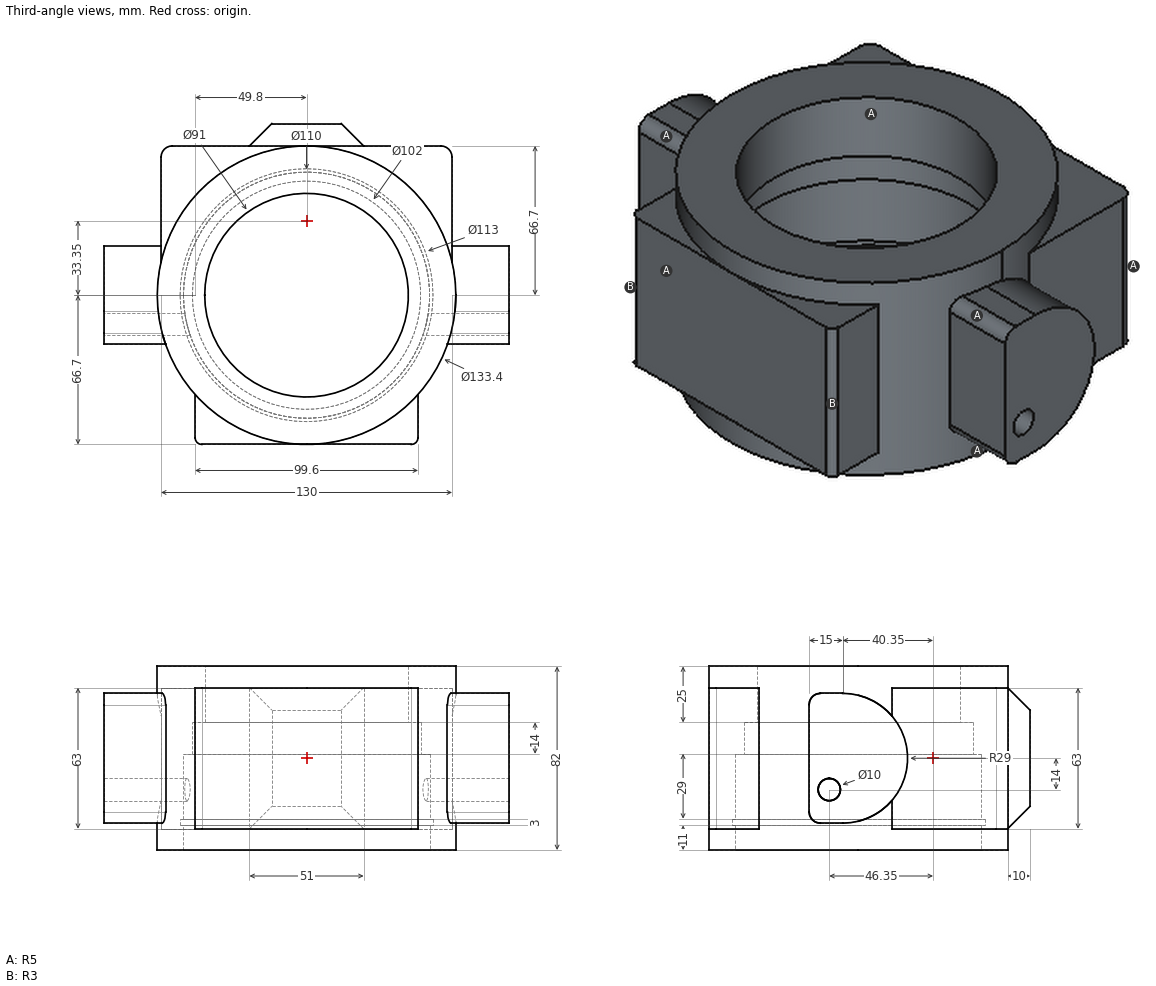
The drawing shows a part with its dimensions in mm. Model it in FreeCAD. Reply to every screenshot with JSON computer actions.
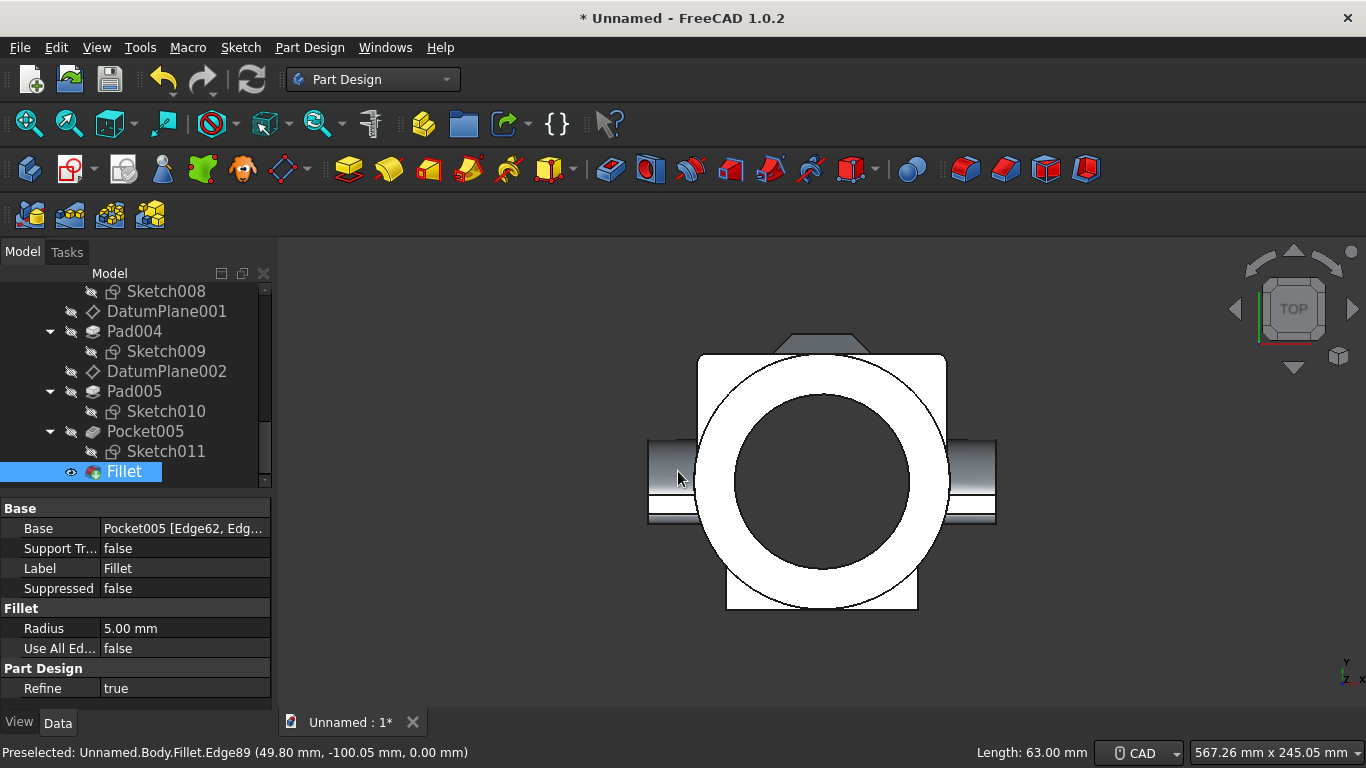
{"action": "key", "text": "1"}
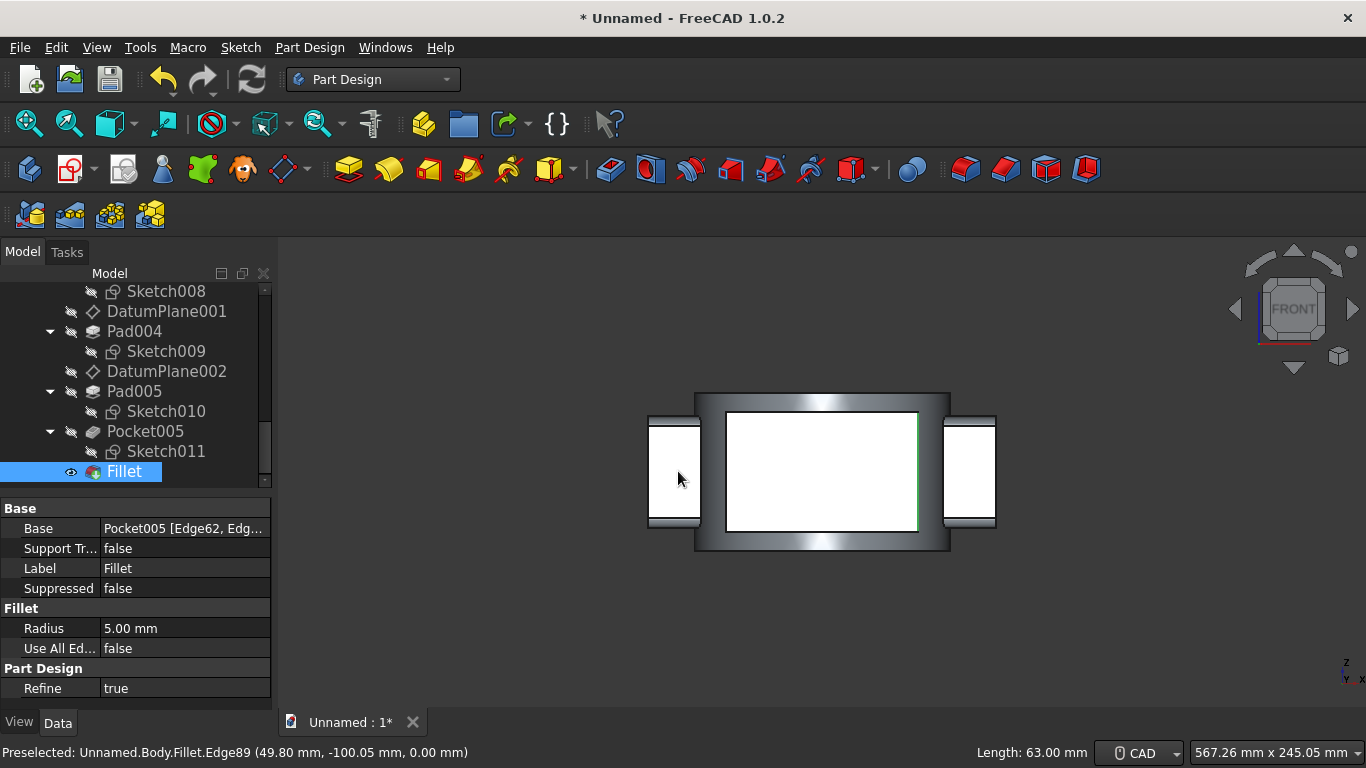
{"action": "left_click", "coordinate": [30, 124]}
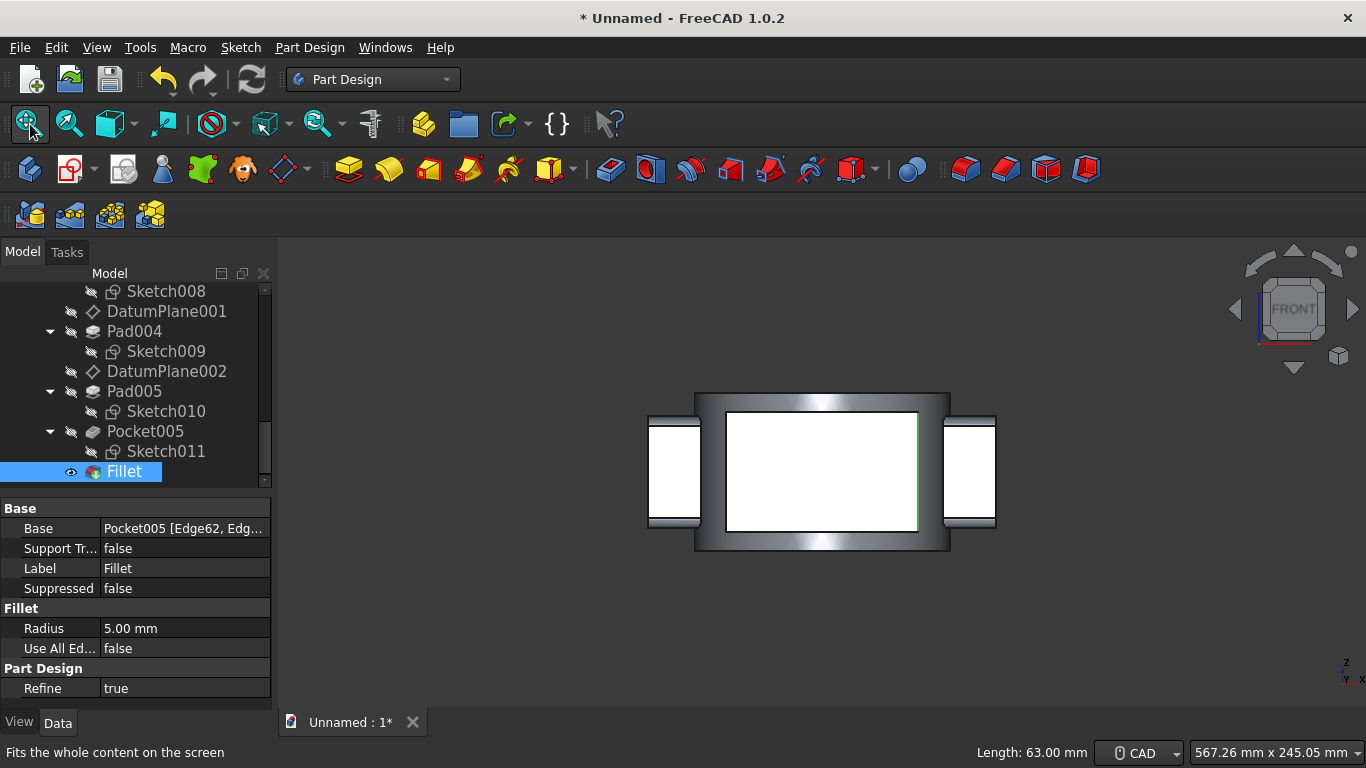
{"action": "left_click", "coordinate": [726, 471], "text": "ctrl"}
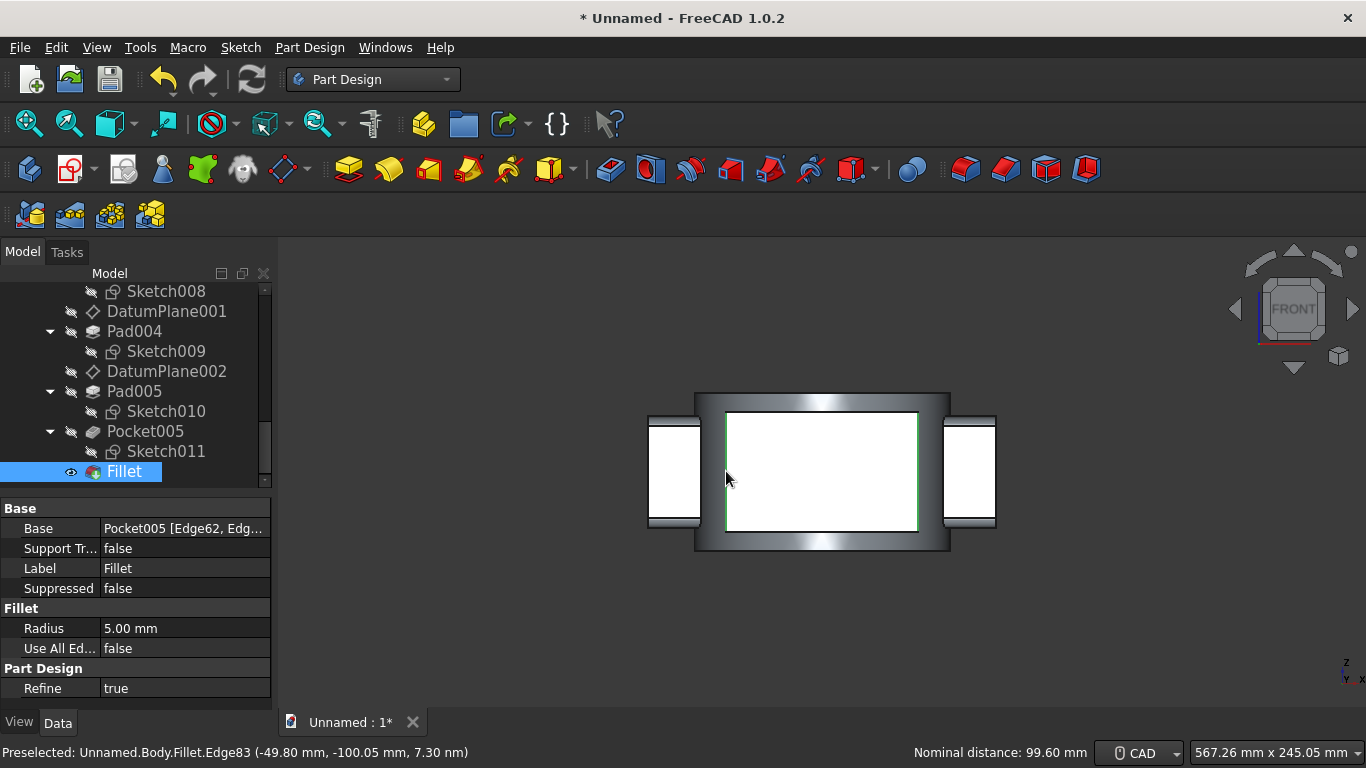
{"action": "left_click", "coordinate": [966, 170]}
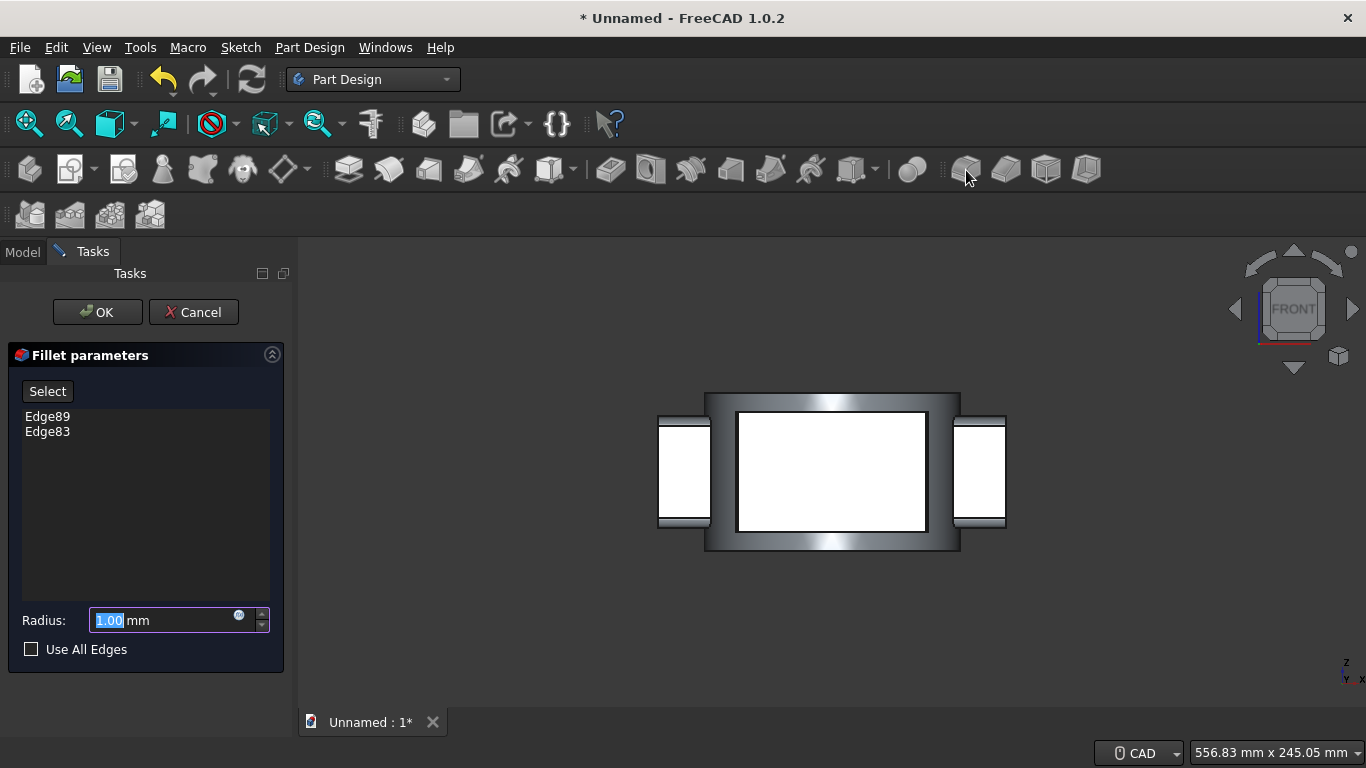
{"action": "type", "text": "3"}
{"action": "key", "text": "Tab"}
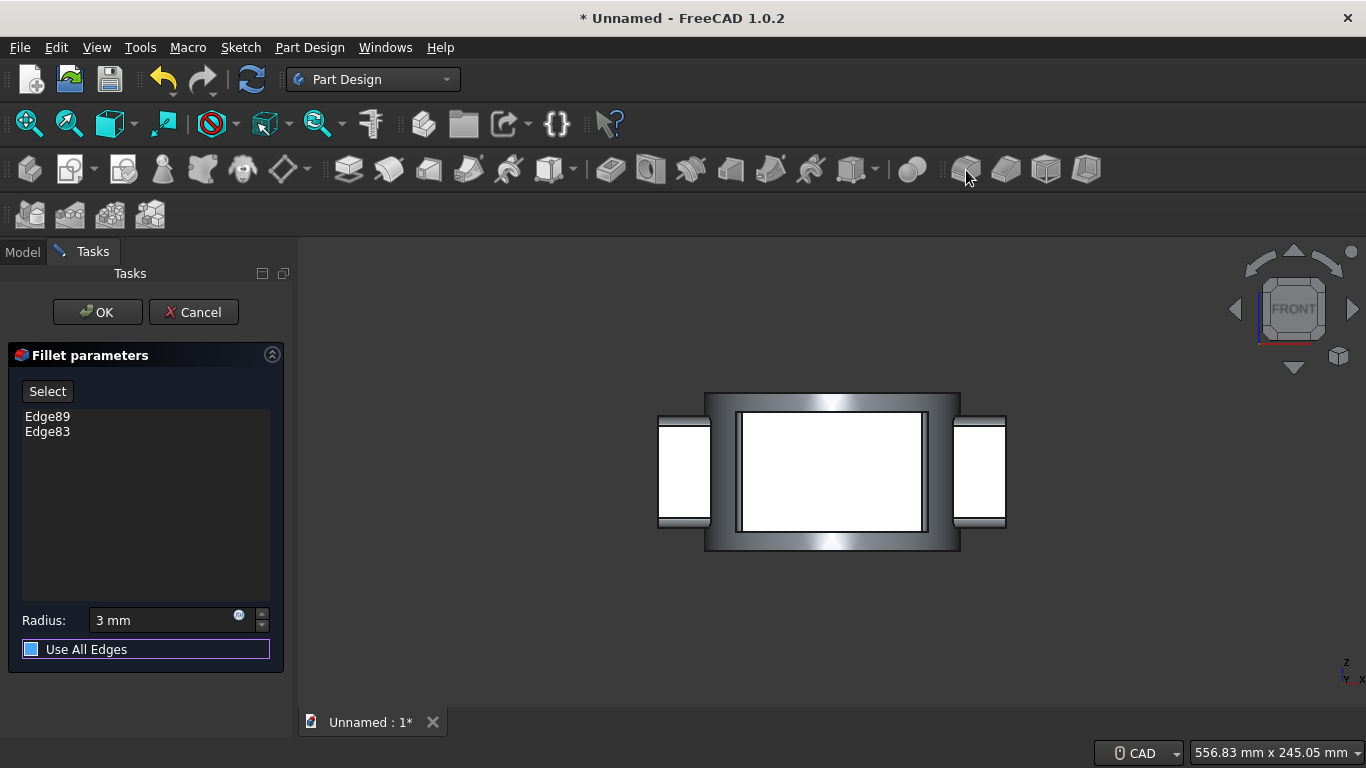
{"action": "left_click", "coordinate": [98, 312]}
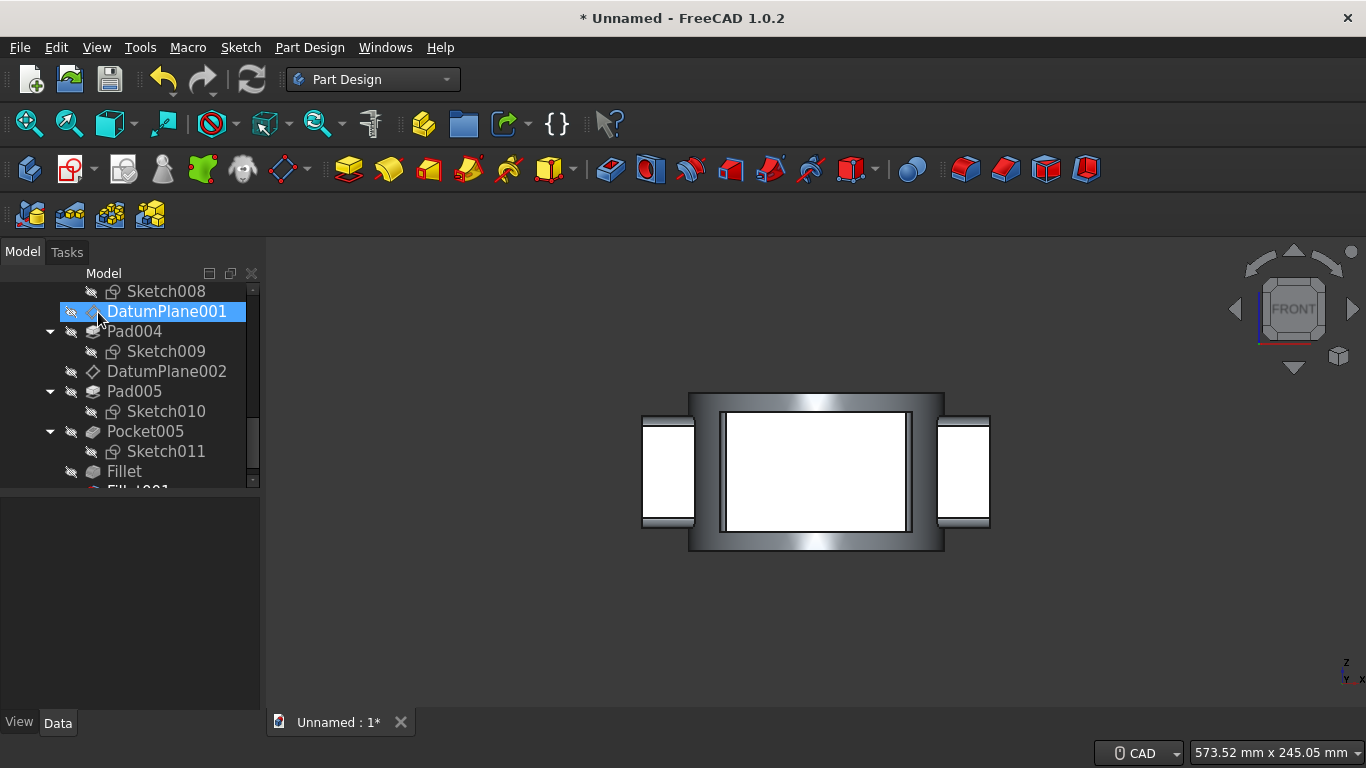
{"action": "key", "text": "0"}